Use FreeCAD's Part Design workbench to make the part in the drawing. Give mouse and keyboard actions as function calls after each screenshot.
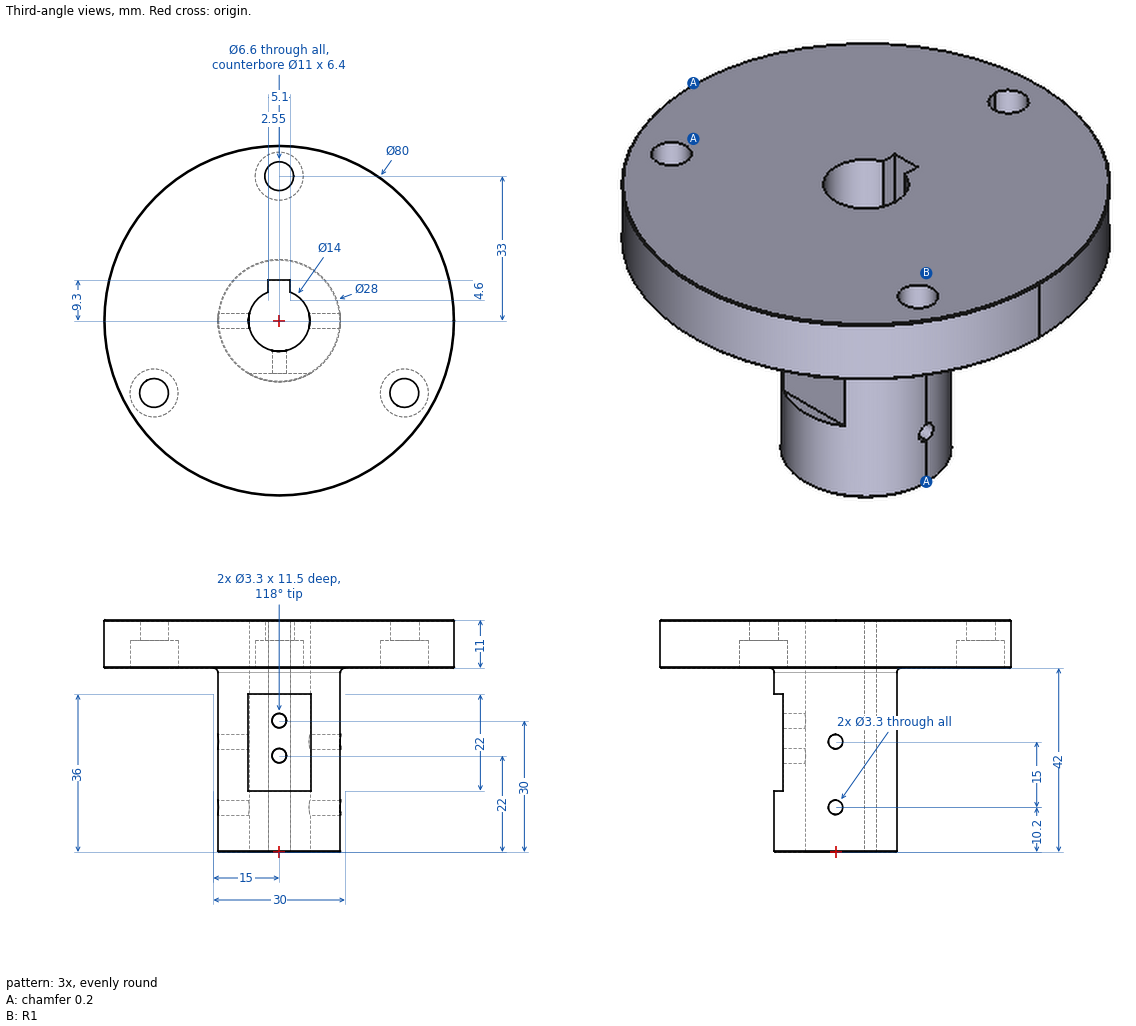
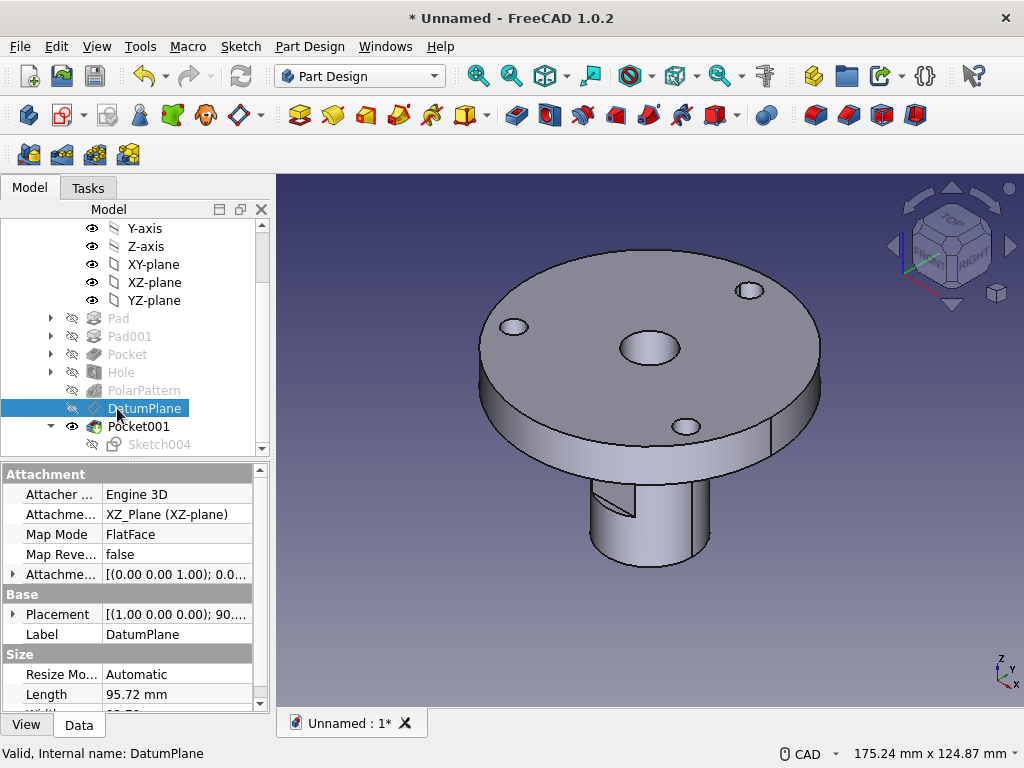
key(1)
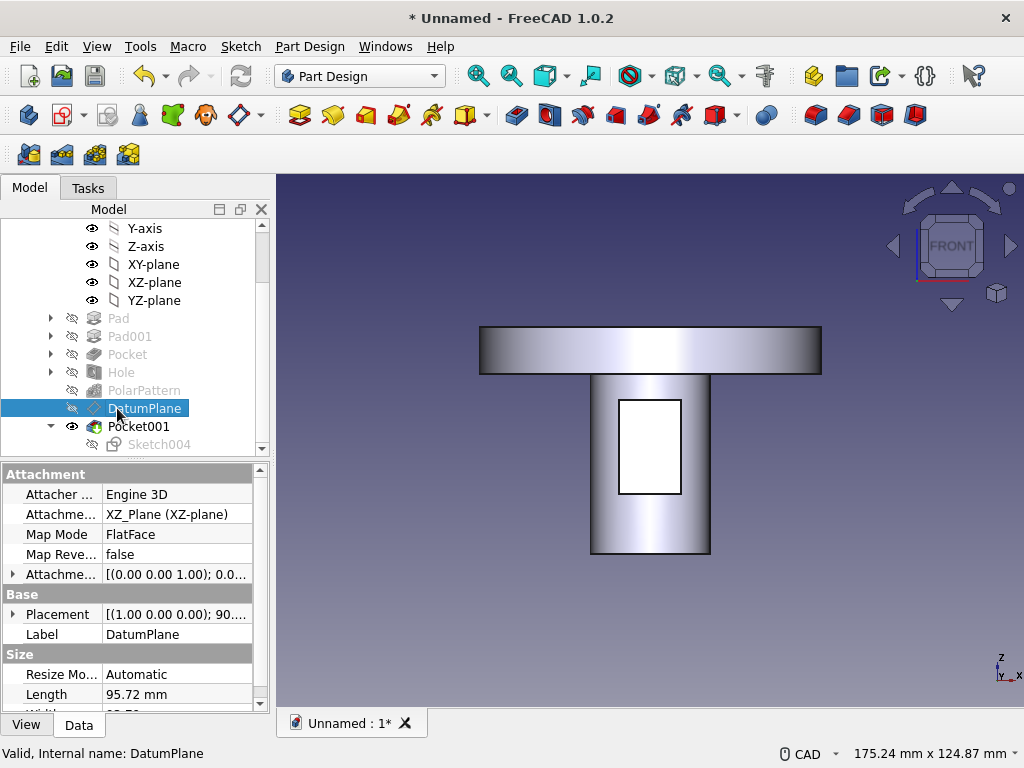
click(650, 432)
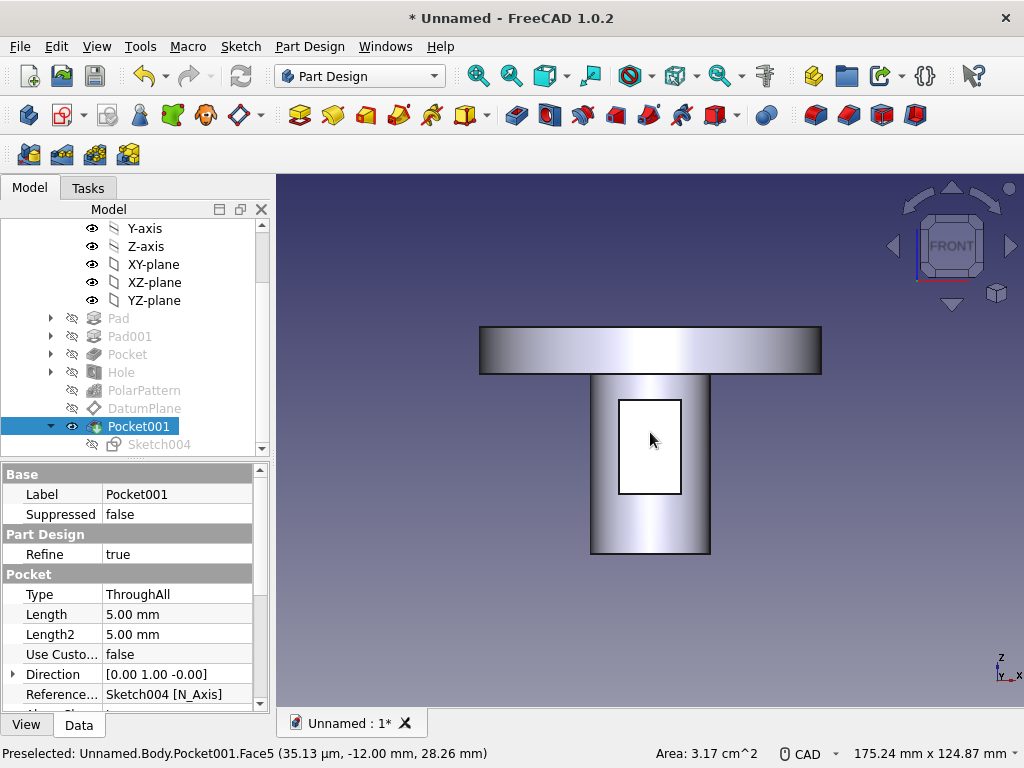
click(62, 116)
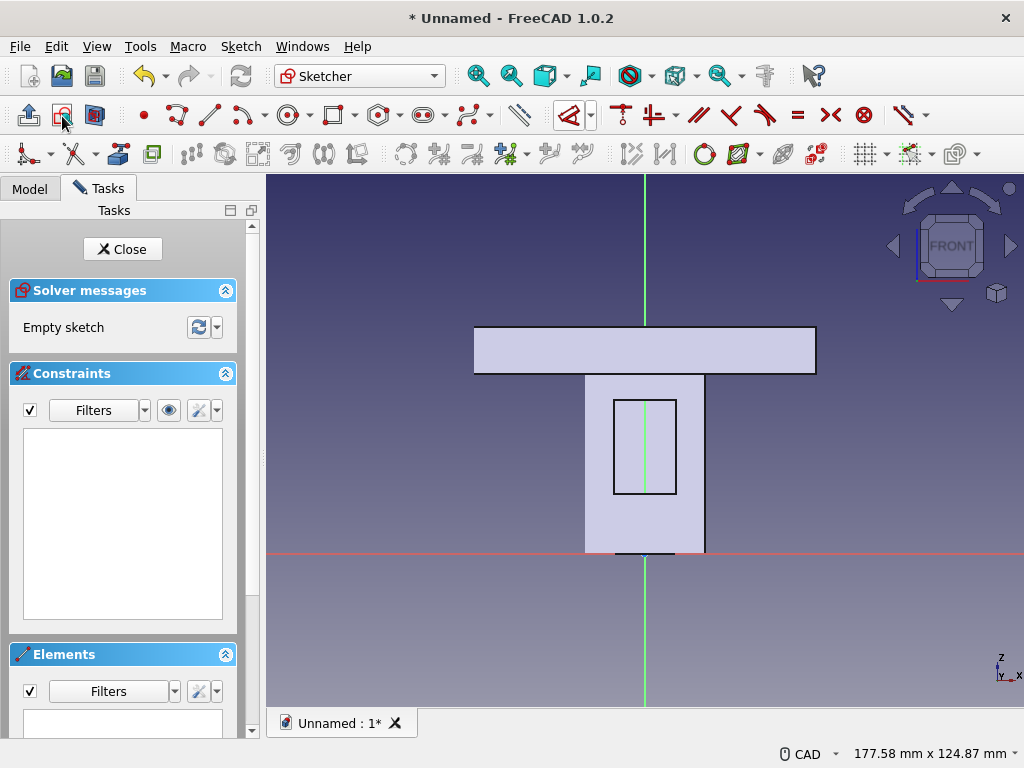
scroll(656, 443, up, 10)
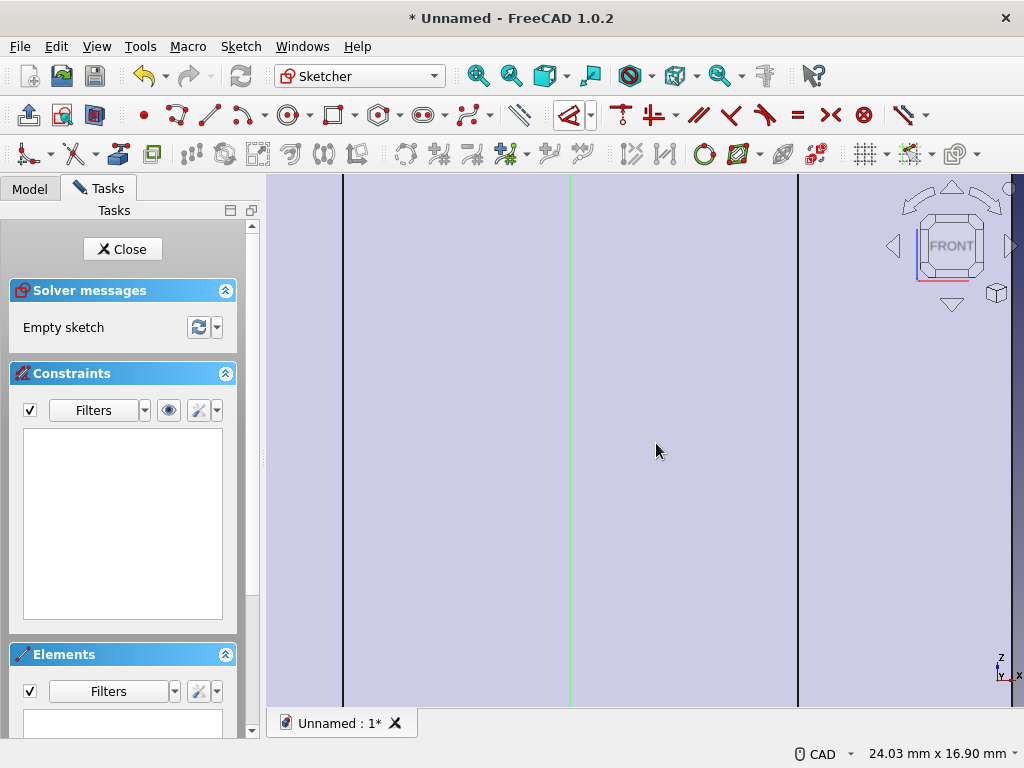
key(g)
key(c)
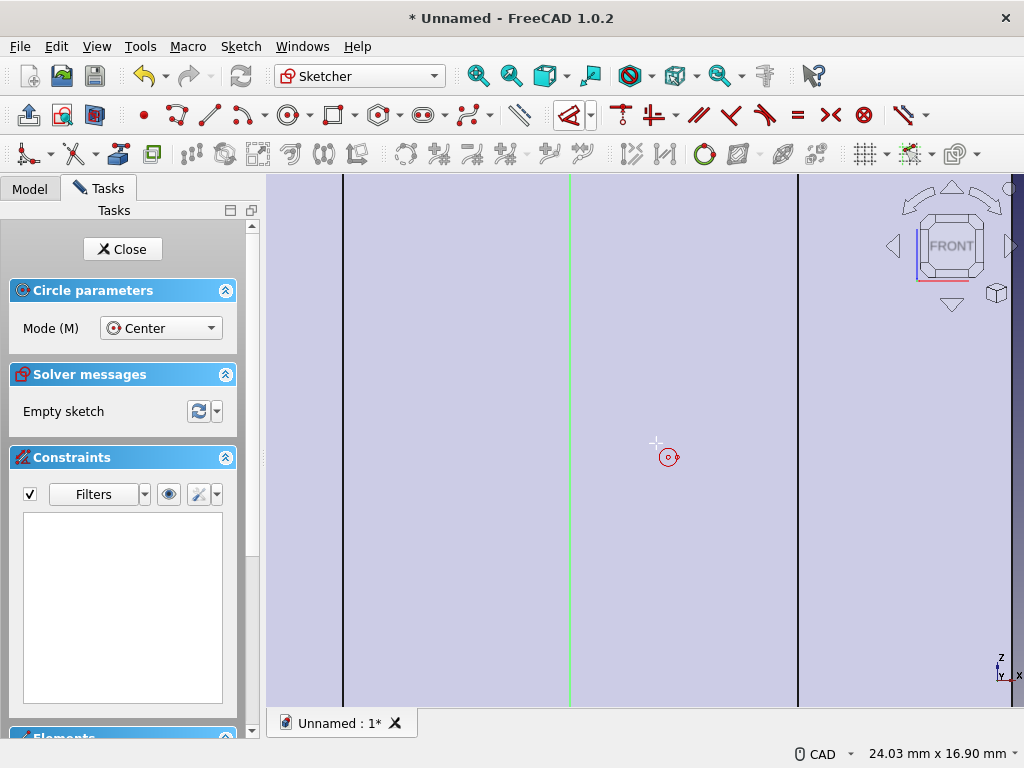
click(570, 311)
move(607, 274)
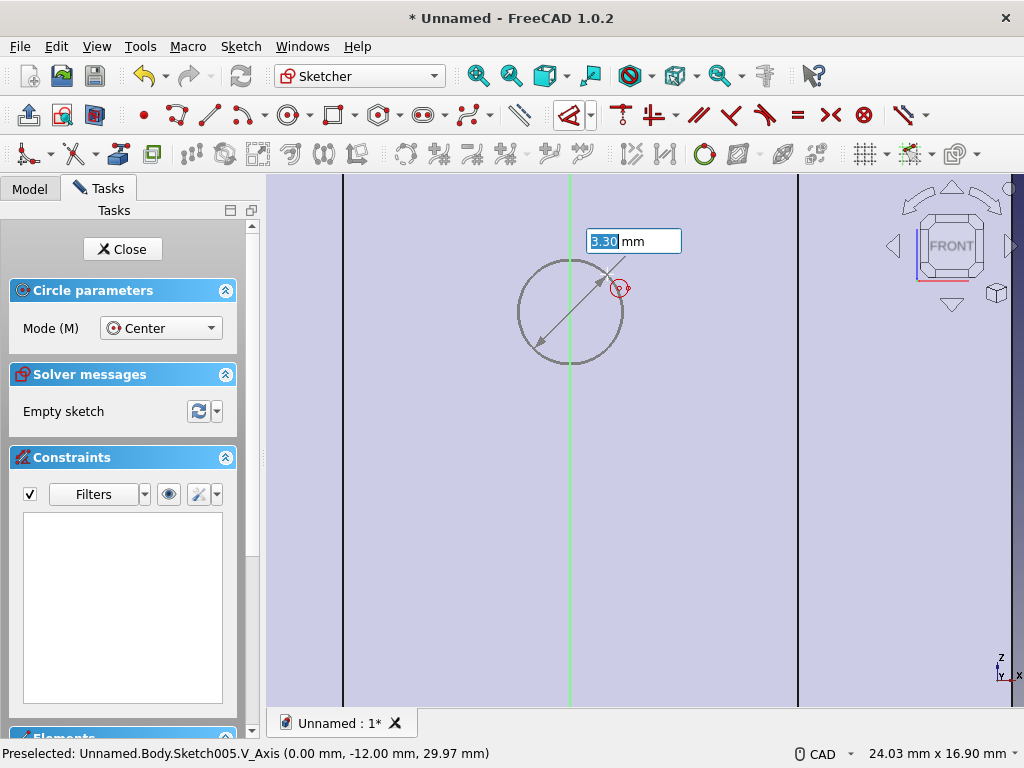
text(3.3)
key(Return)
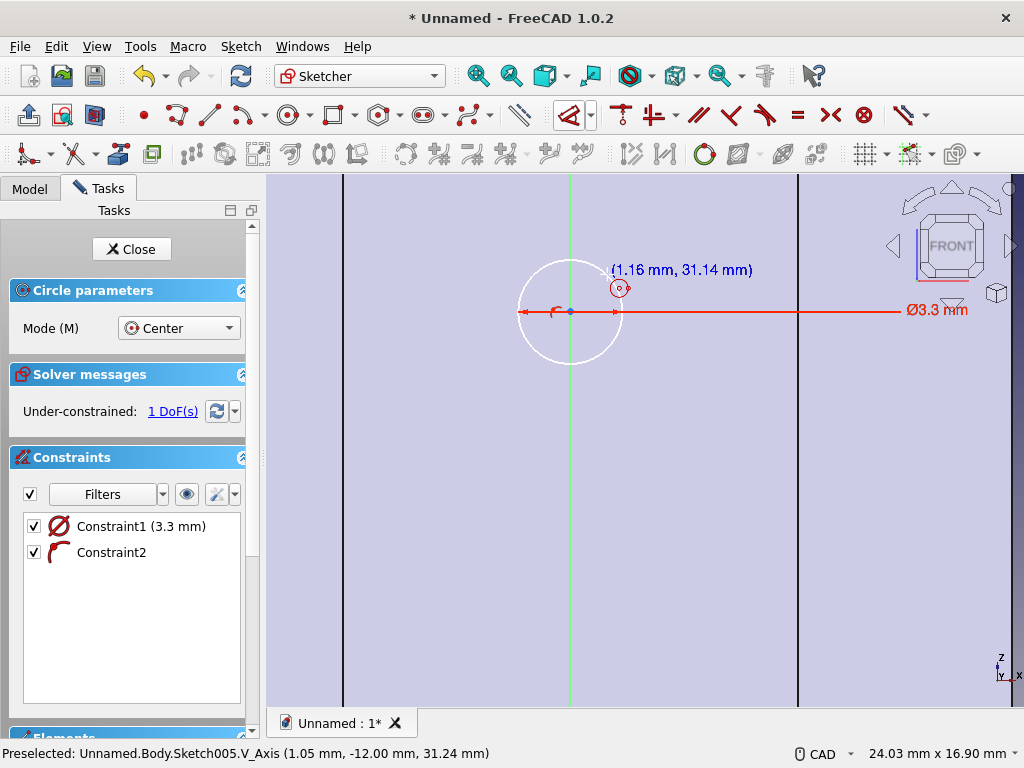
click(570, 563)
move(607, 526)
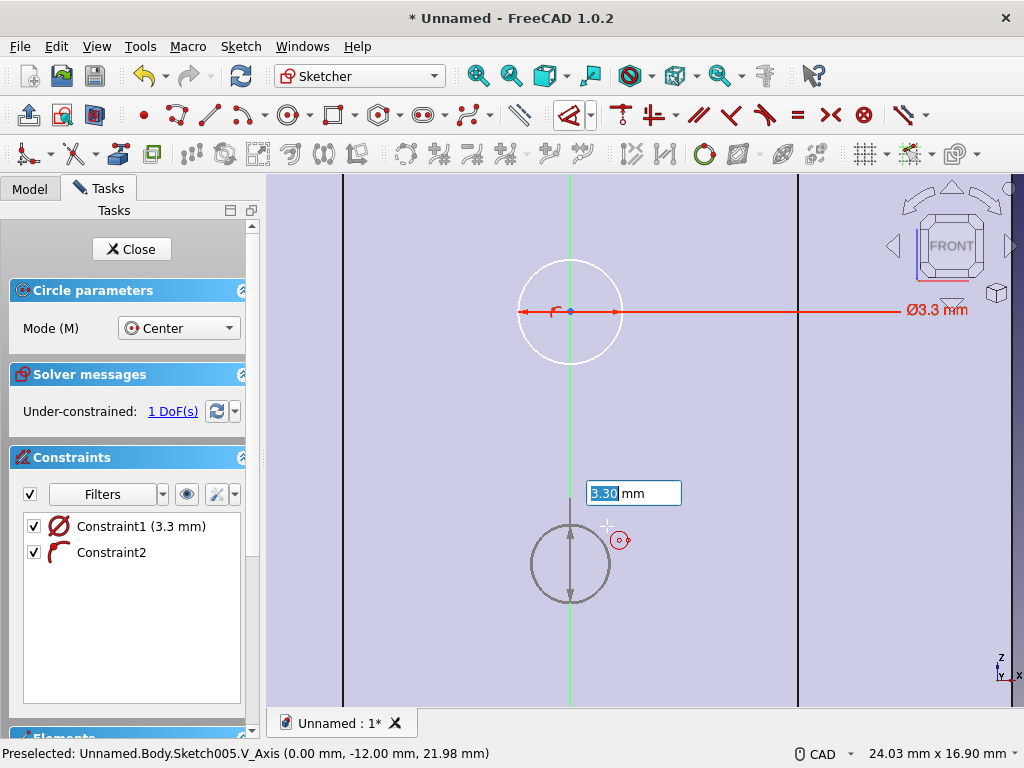
text(3.3)
key(Return)
key(Escape)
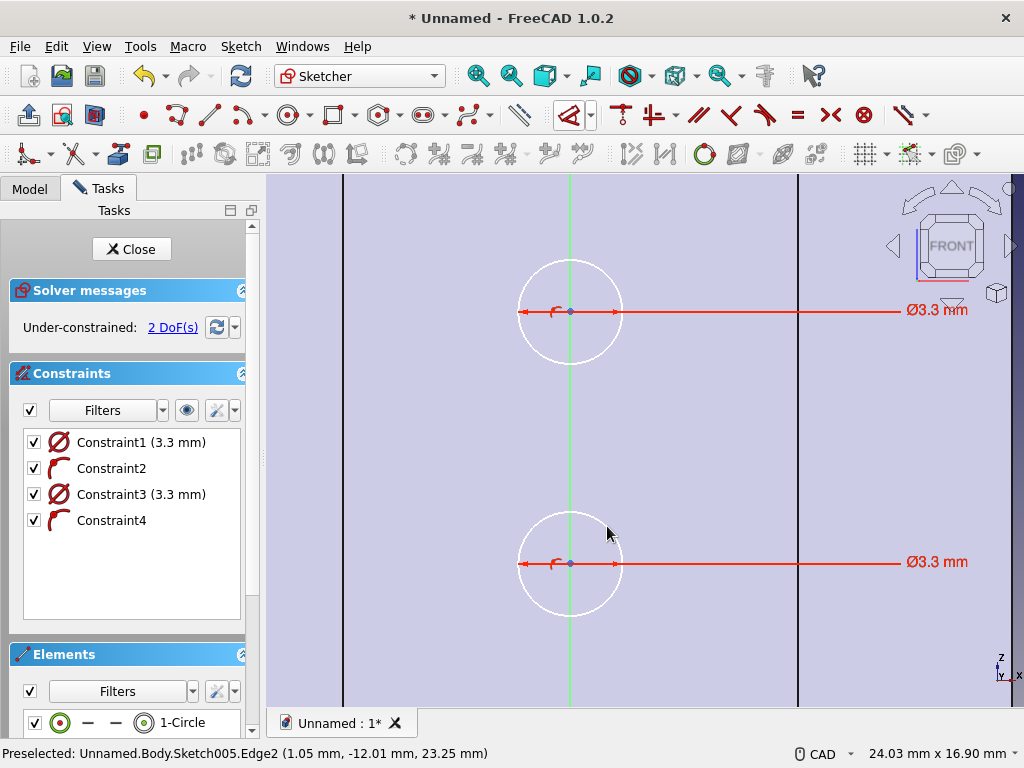
click(570, 312)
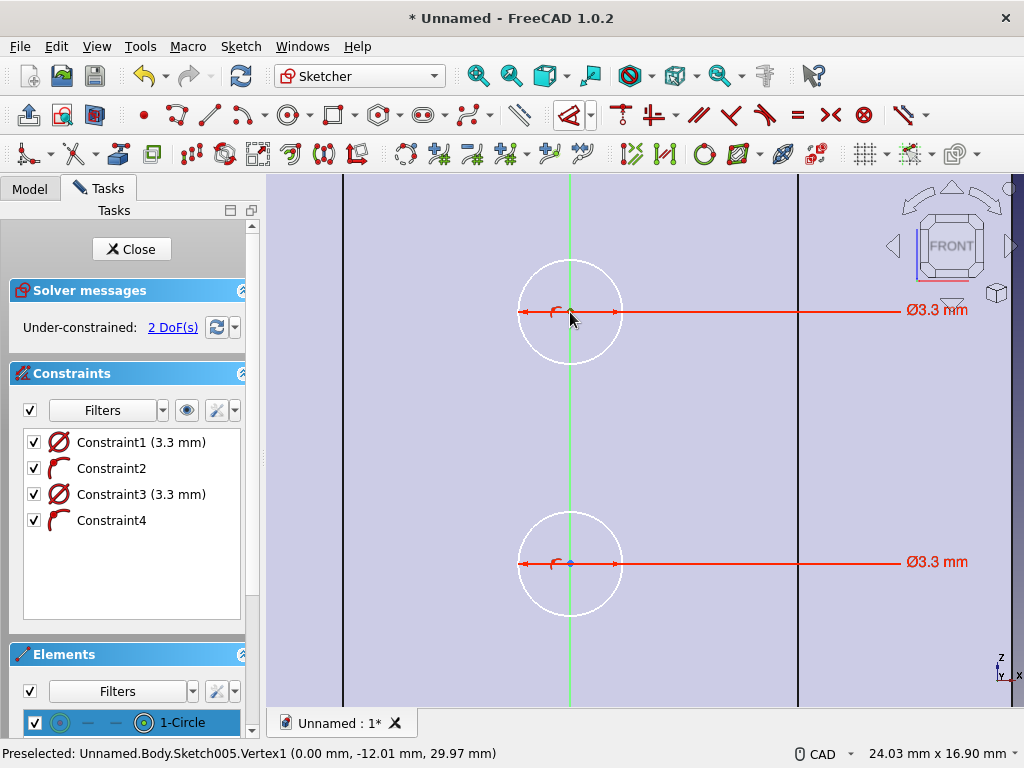
key(i)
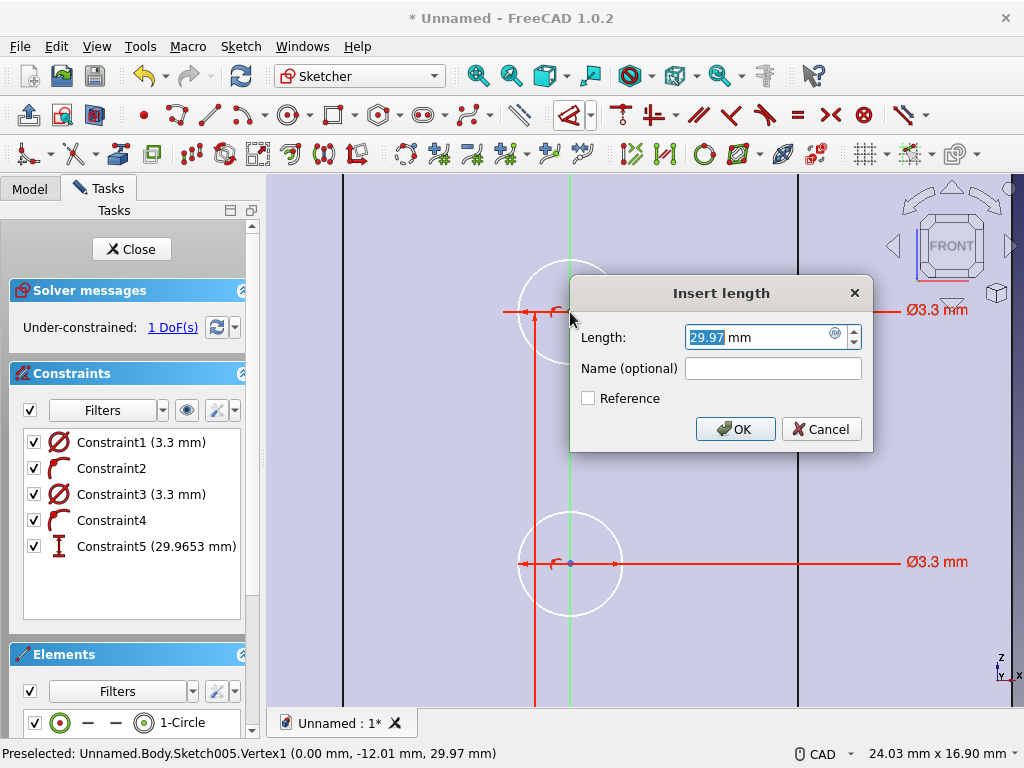
text(30)
key(Return)